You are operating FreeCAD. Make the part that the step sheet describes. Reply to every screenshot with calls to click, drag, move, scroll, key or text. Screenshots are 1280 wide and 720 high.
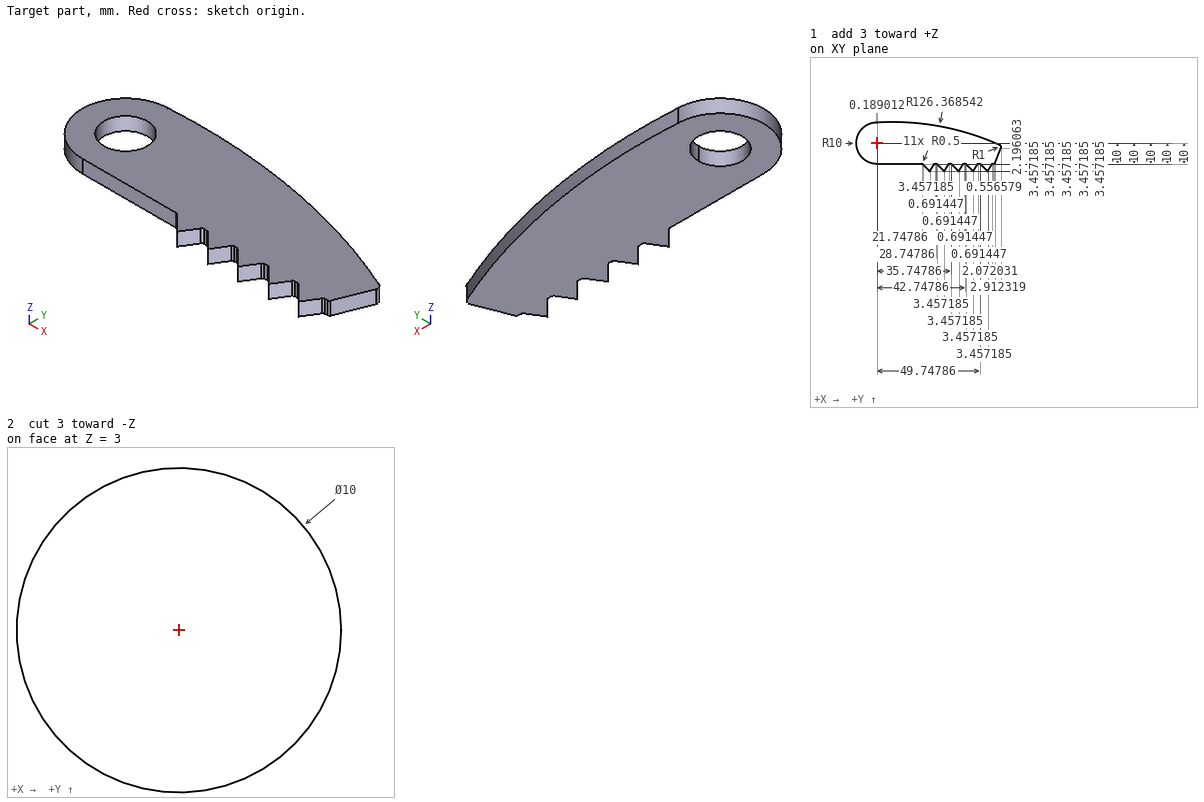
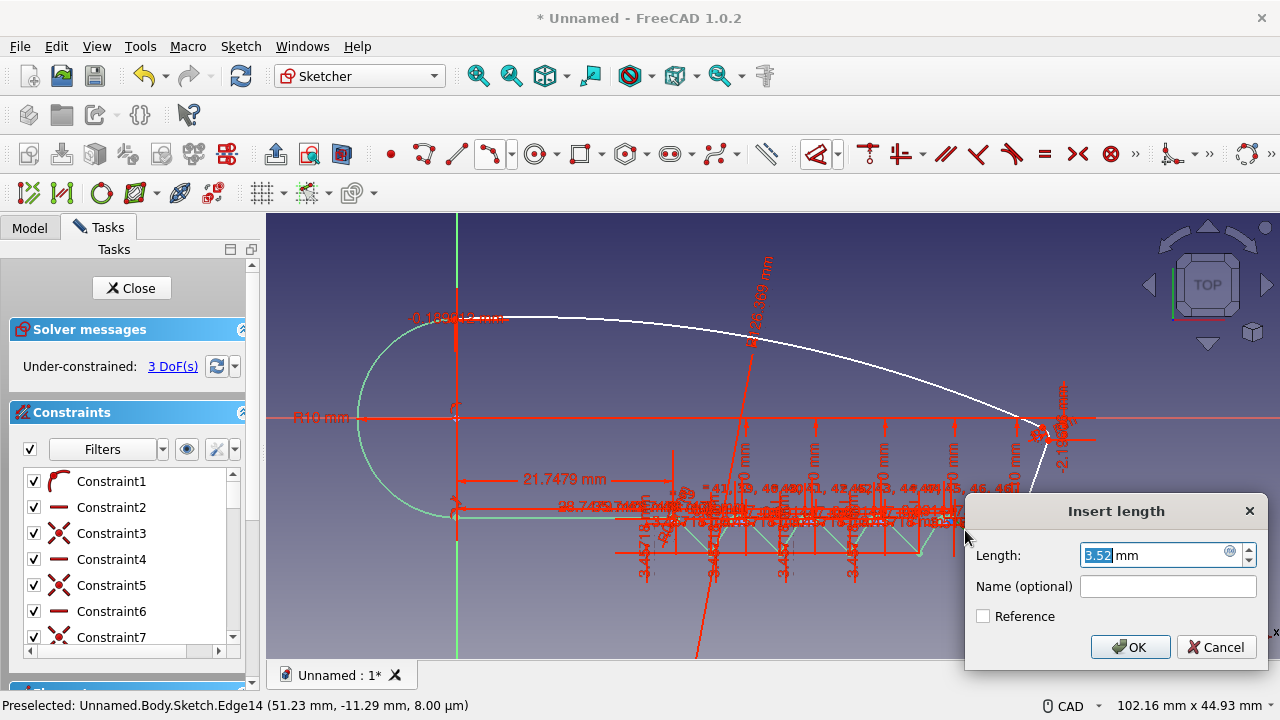
text(3.457185)
key(Return)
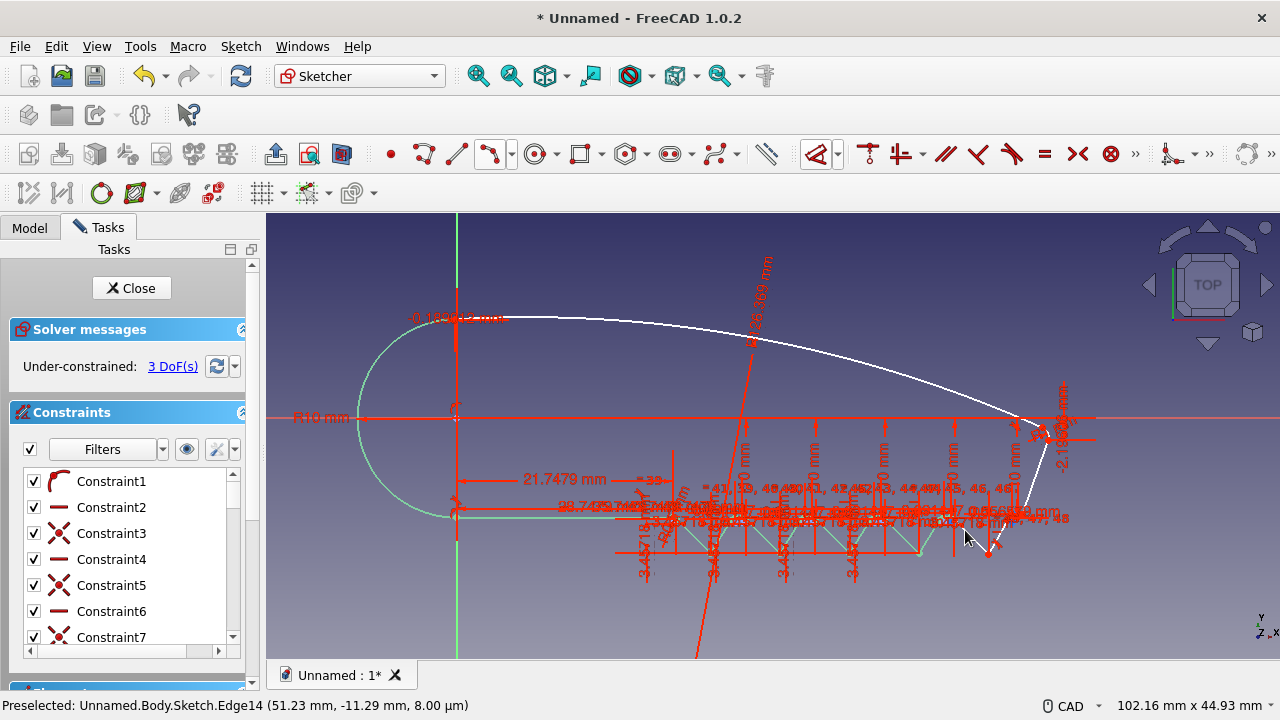
click(978, 544)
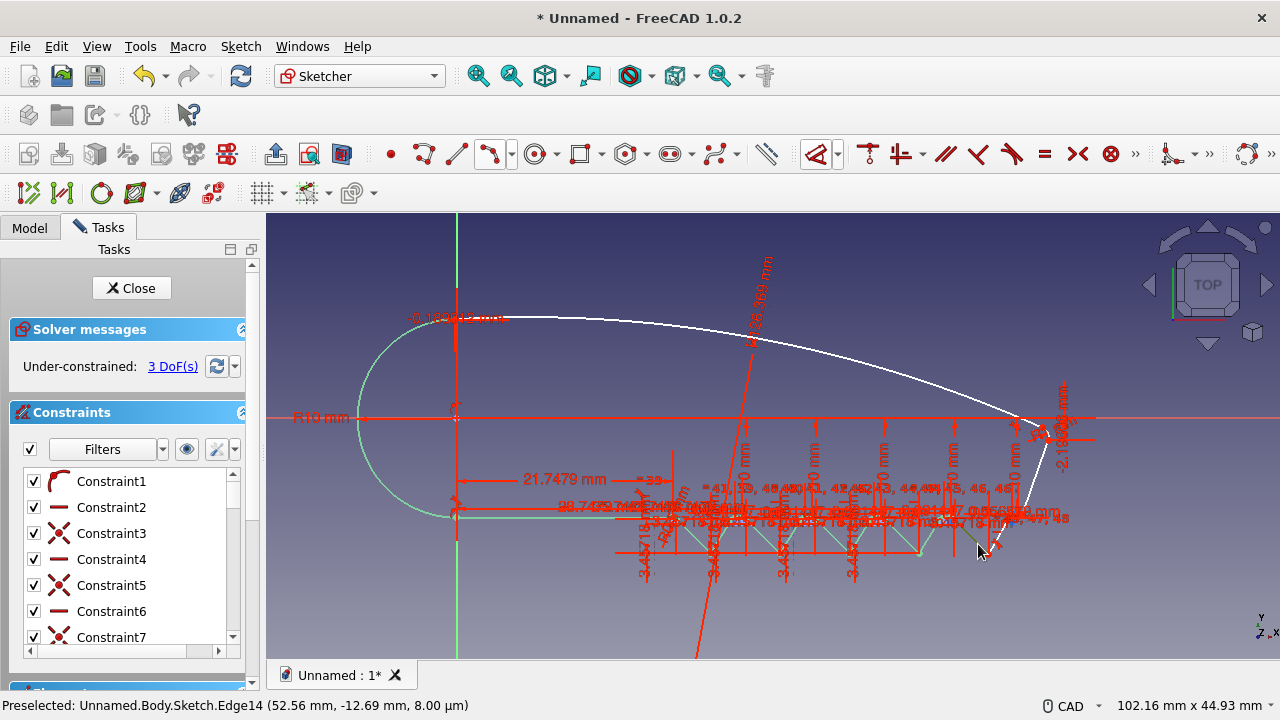
click(838, 154)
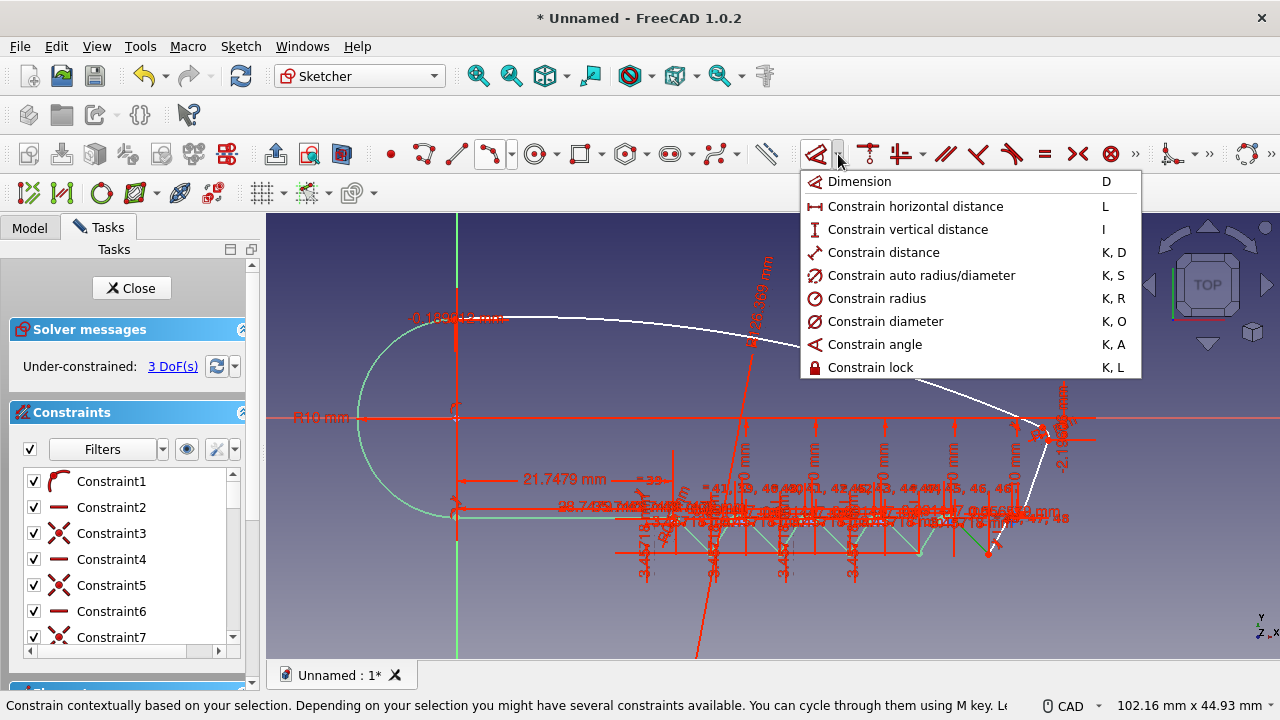
click(971, 230)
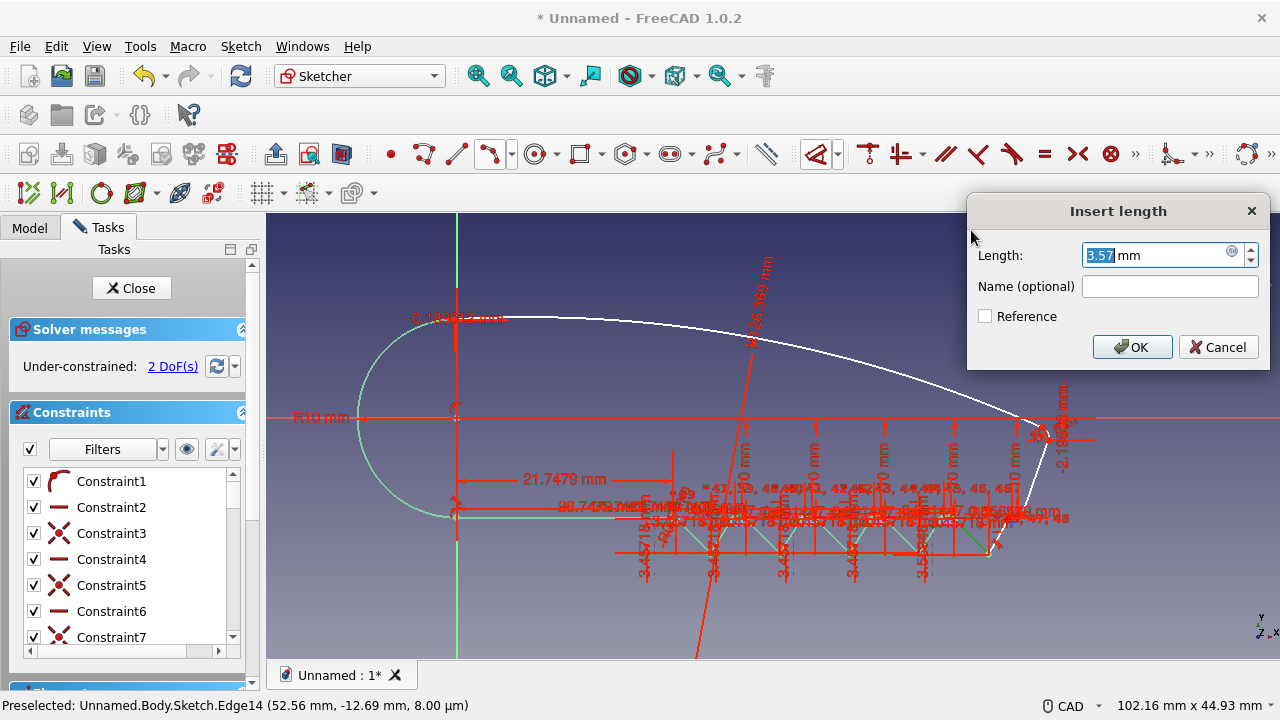
text(3.457185)
key(Return)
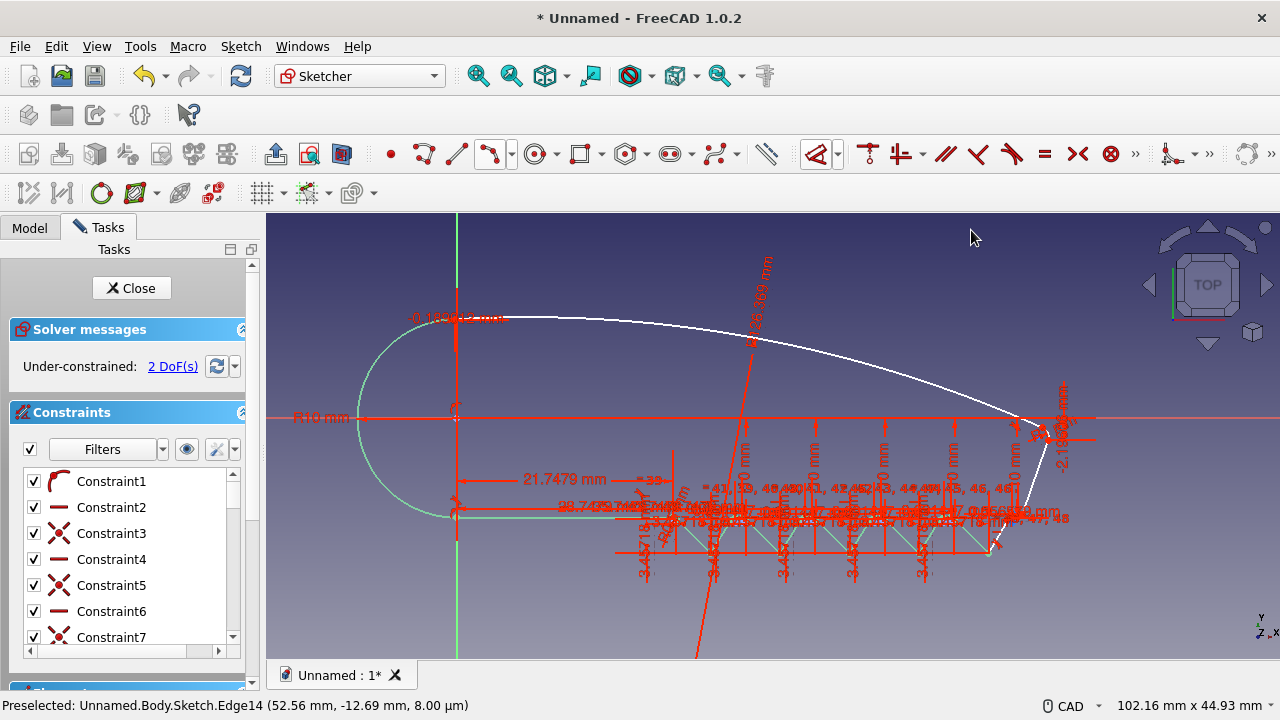
scroll(994, 543, up, 4)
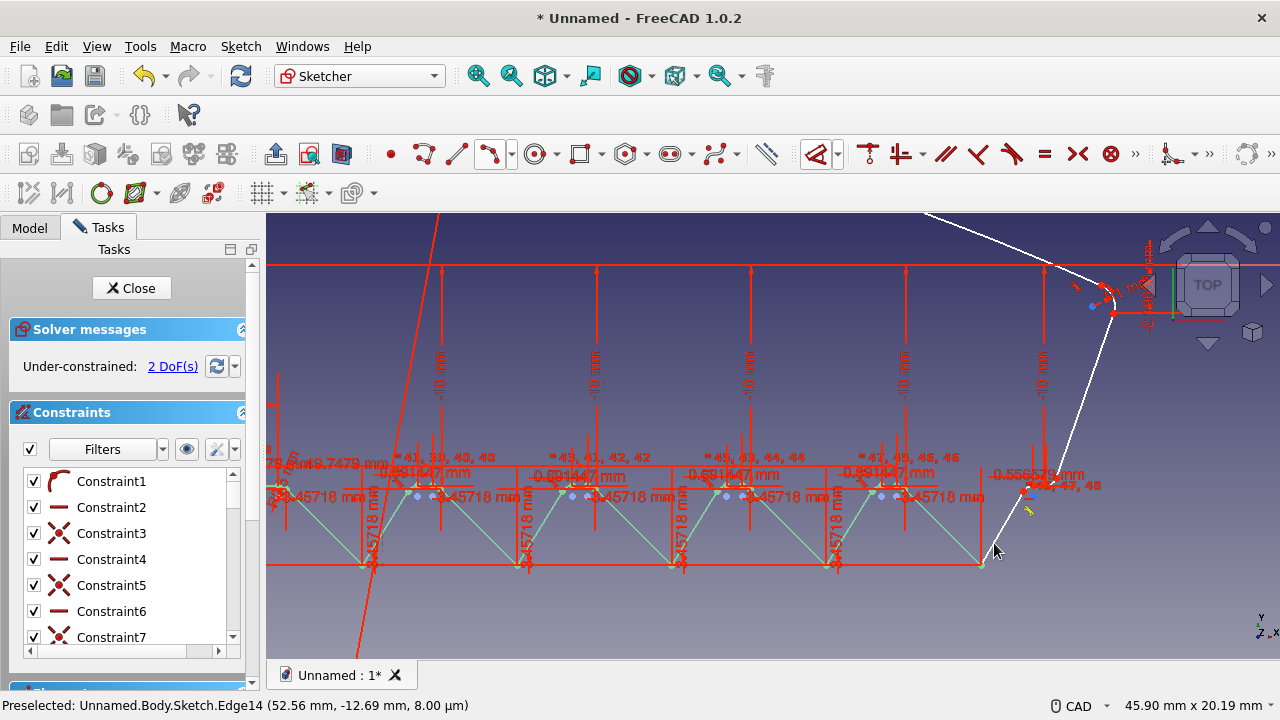
click(994, 543)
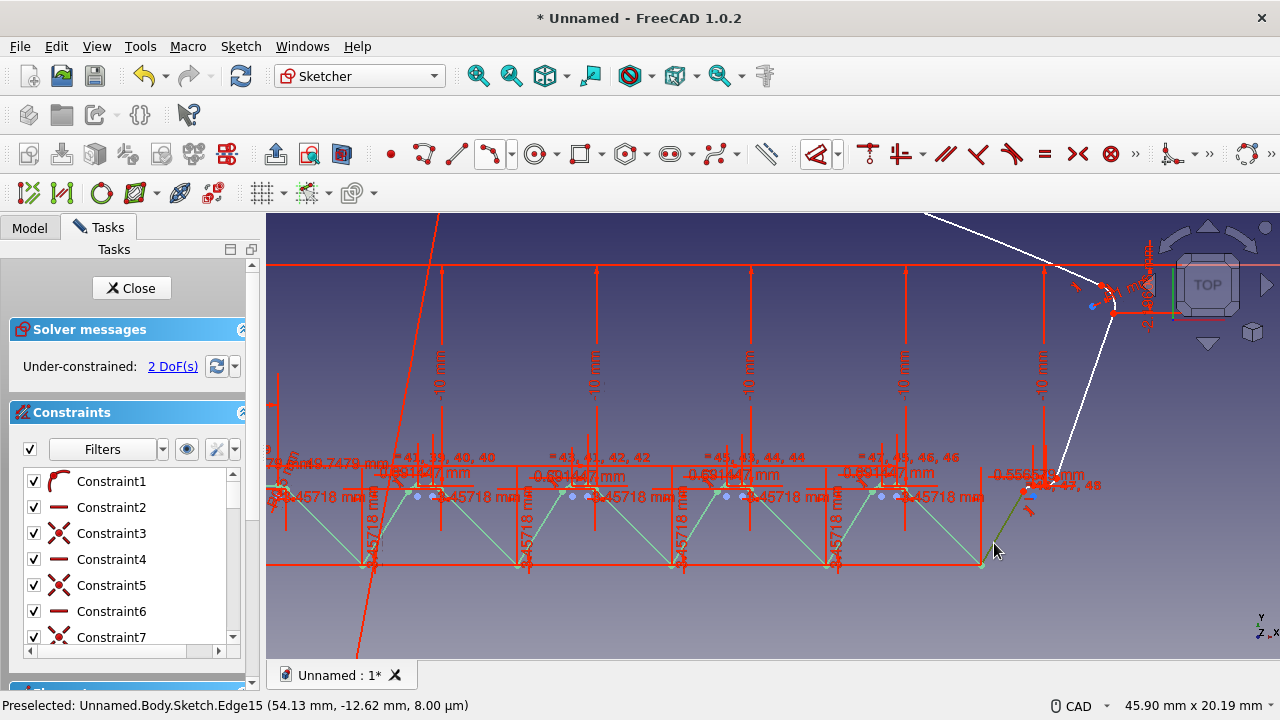
key(l)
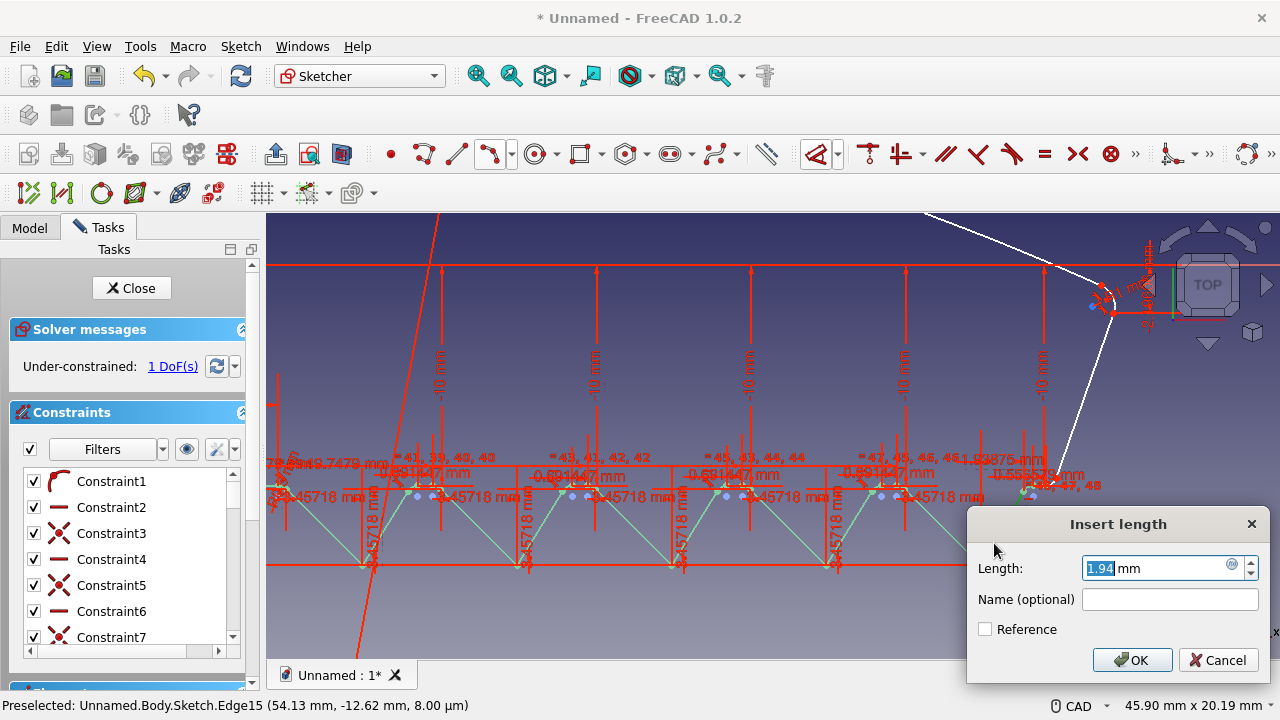
text(2.072031)
key(Return)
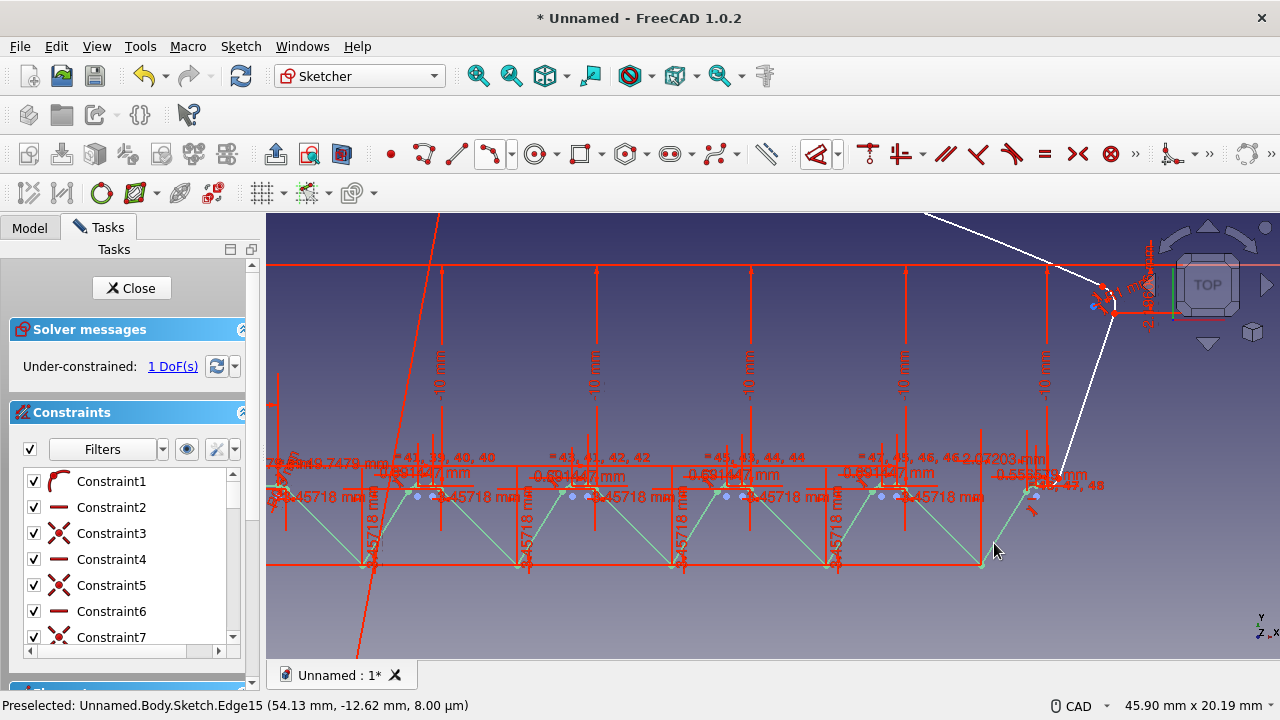
click(1076, 429)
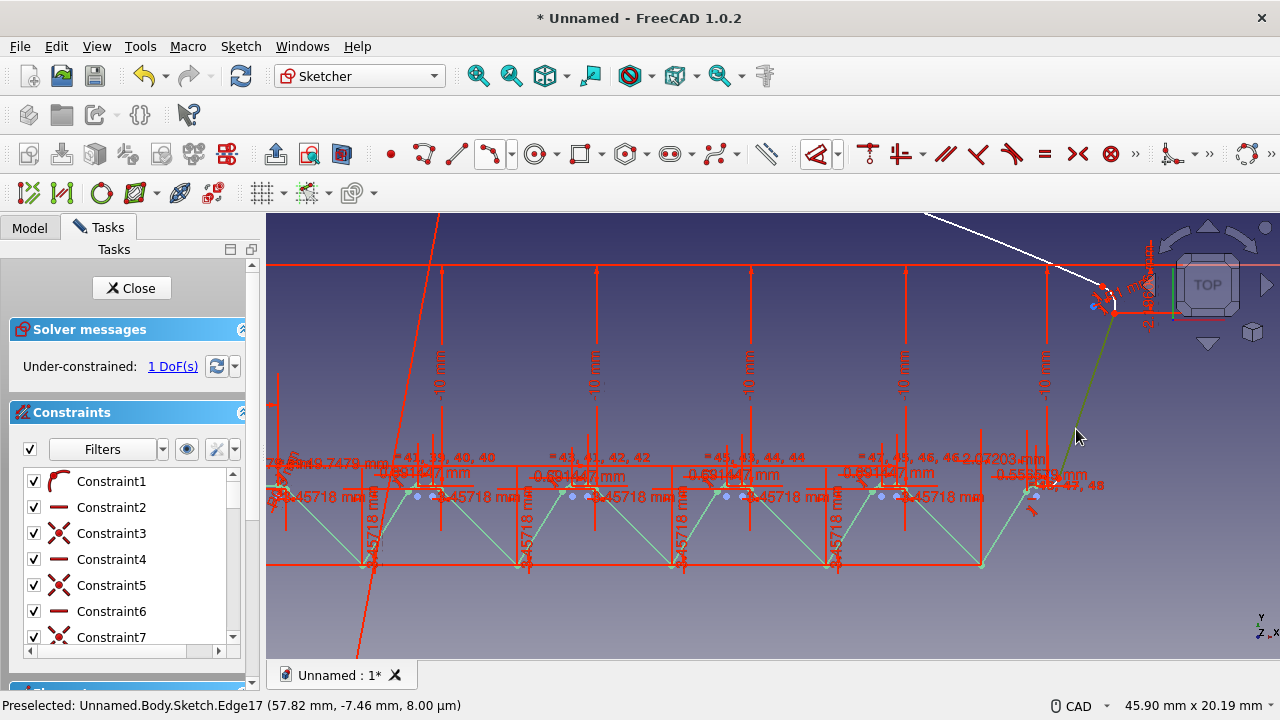
key(l)